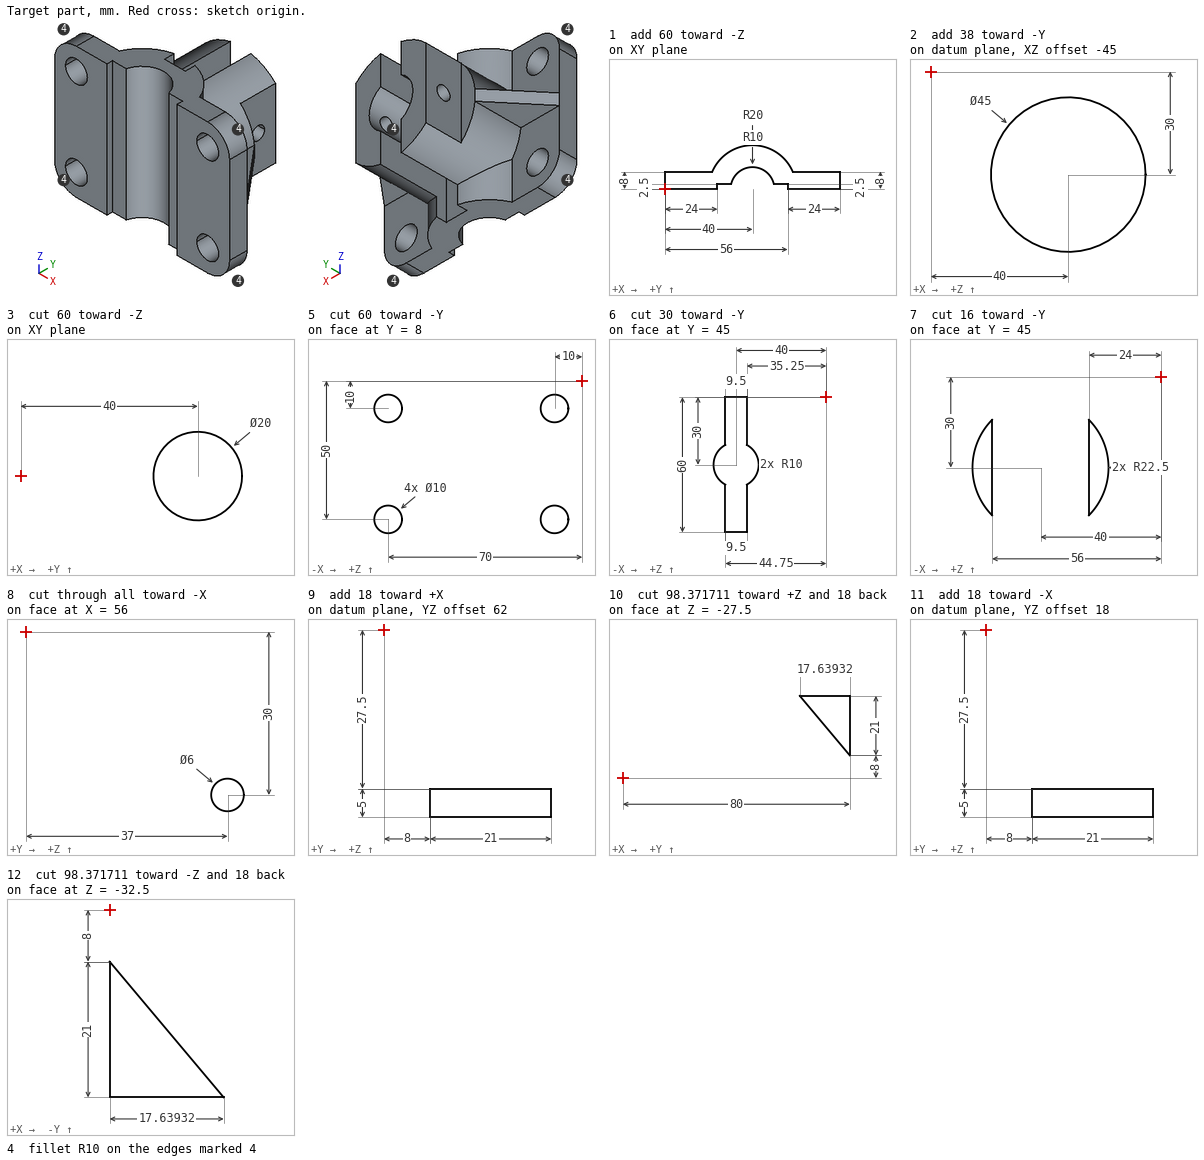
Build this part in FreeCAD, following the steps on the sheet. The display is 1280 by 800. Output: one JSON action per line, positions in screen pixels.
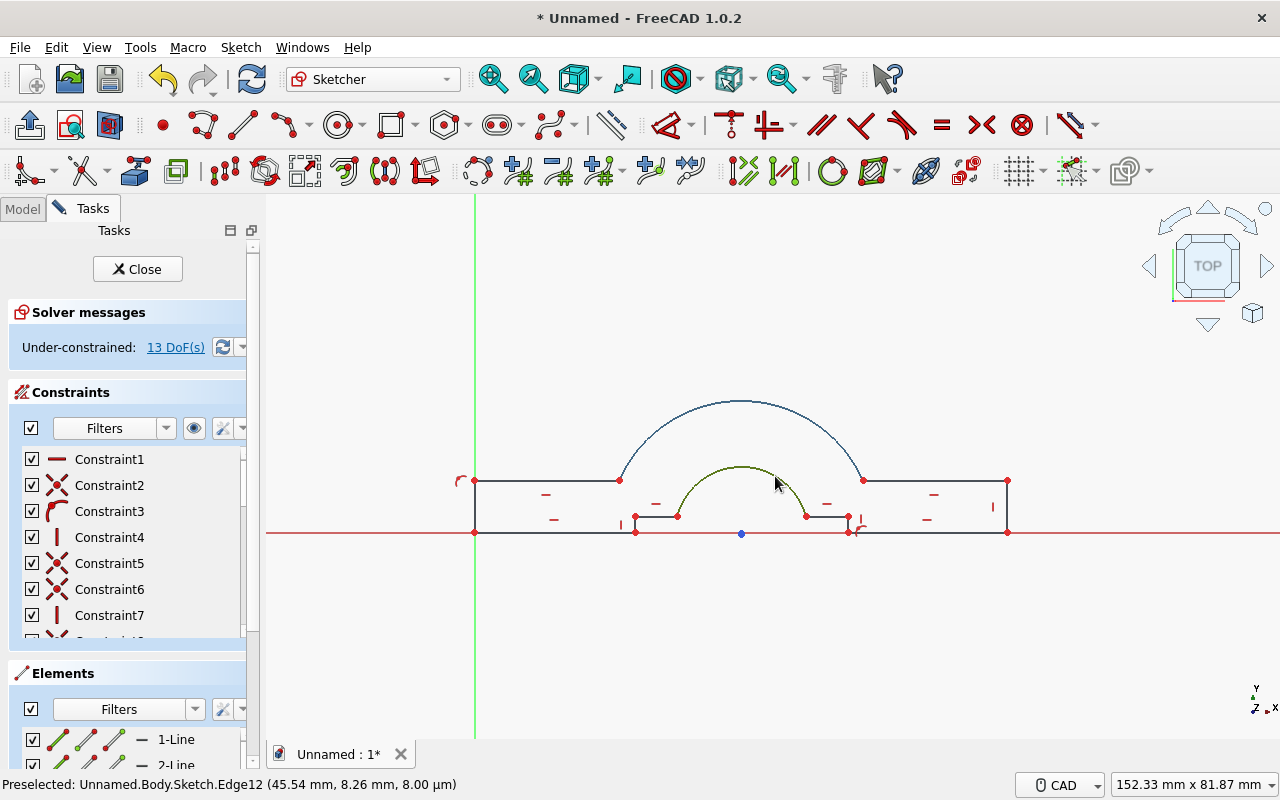
{"action": "left_click", "coordinate": [730, 126]}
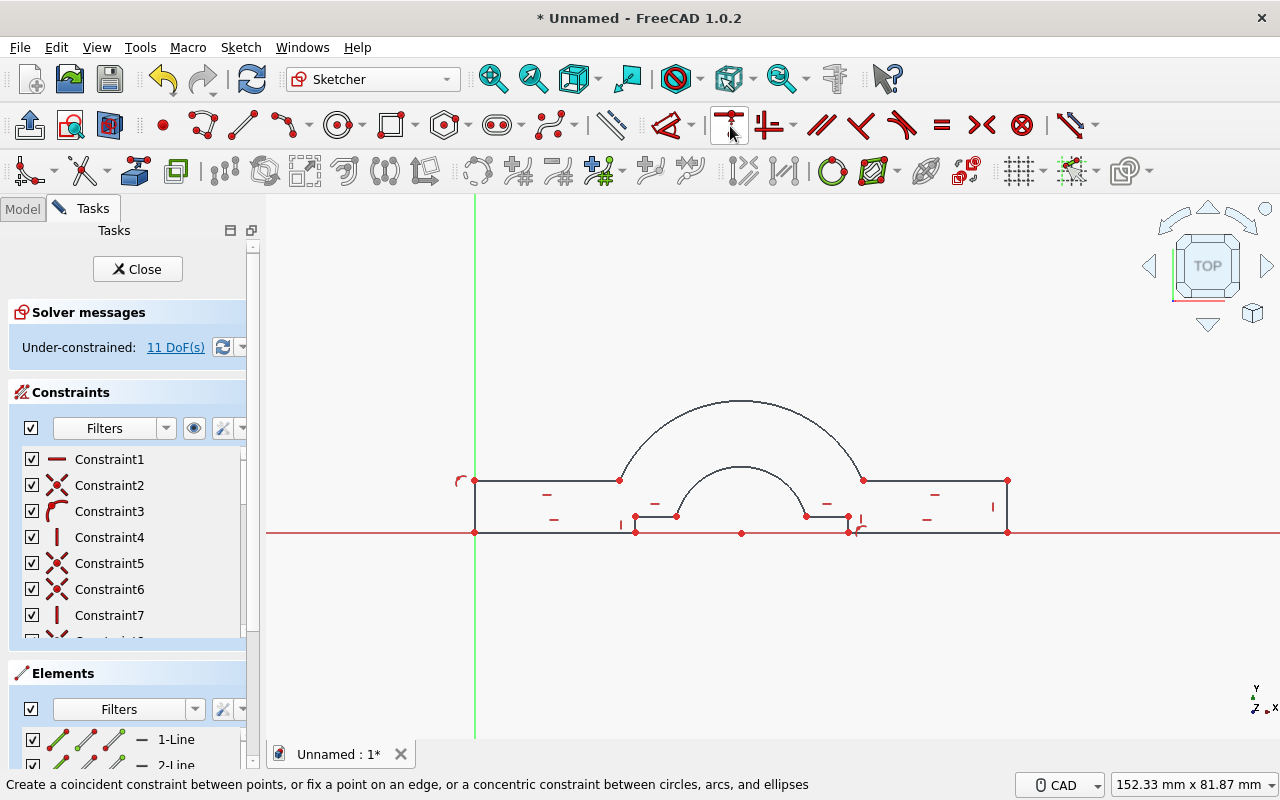
{"action": "left_click", "coordinate": [741, 534]}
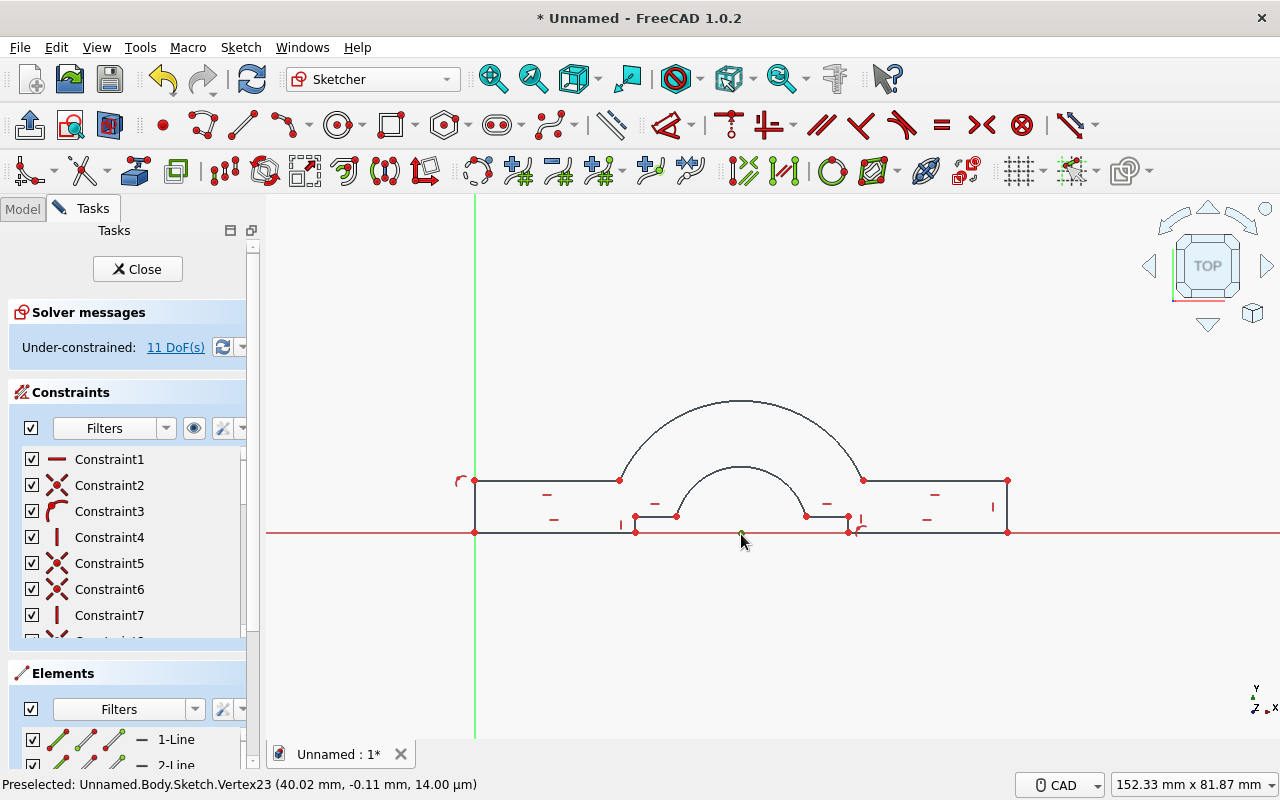
{"action": "left_click", "coordinate": [353, 533]}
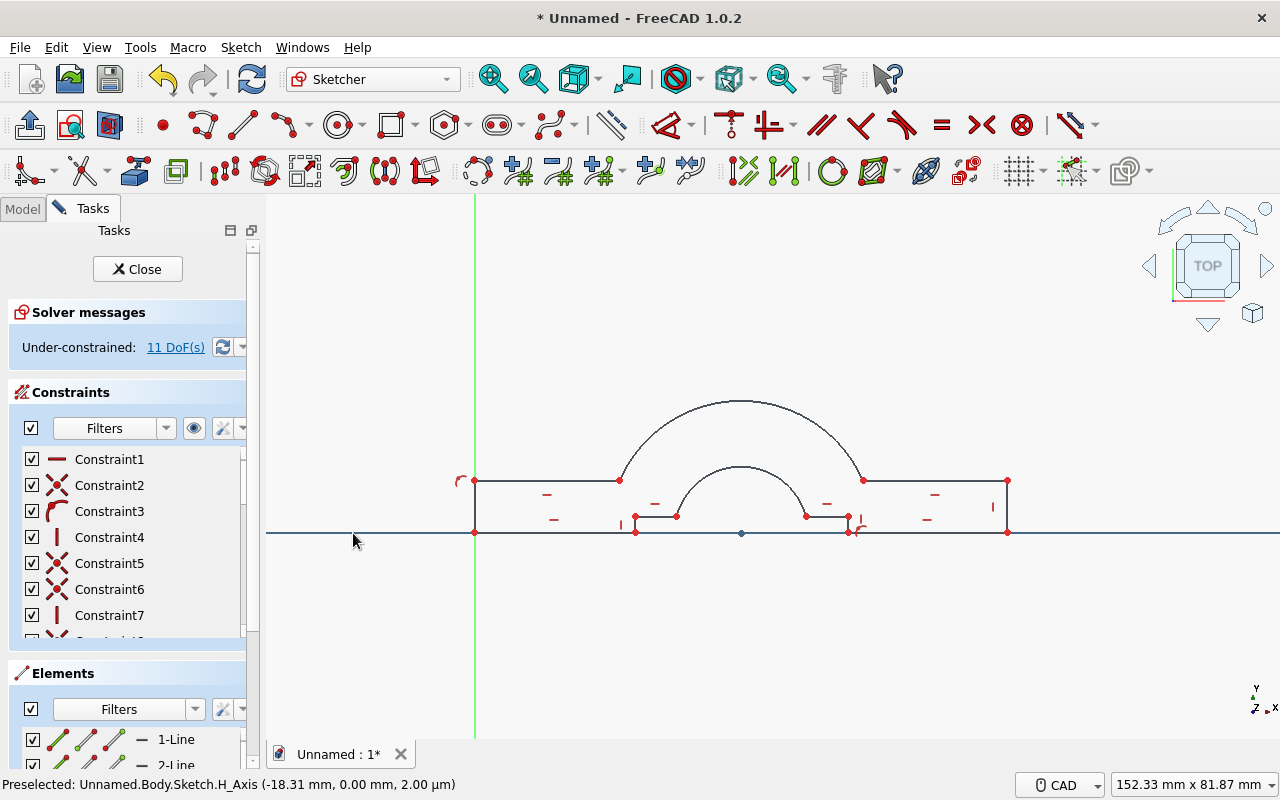
{"action": "left_click", "coordinate": [730, 126]}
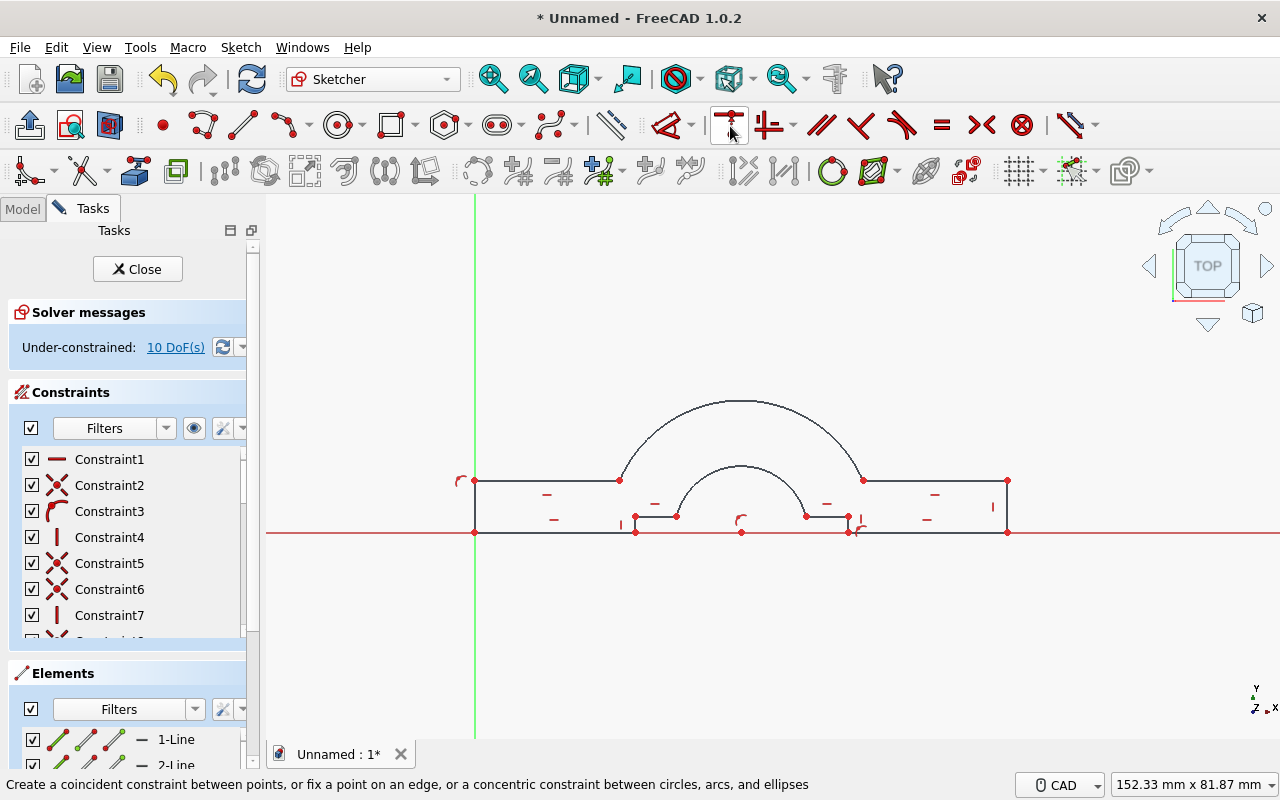
{"action": "left_click", "coordinate": [666, 126]}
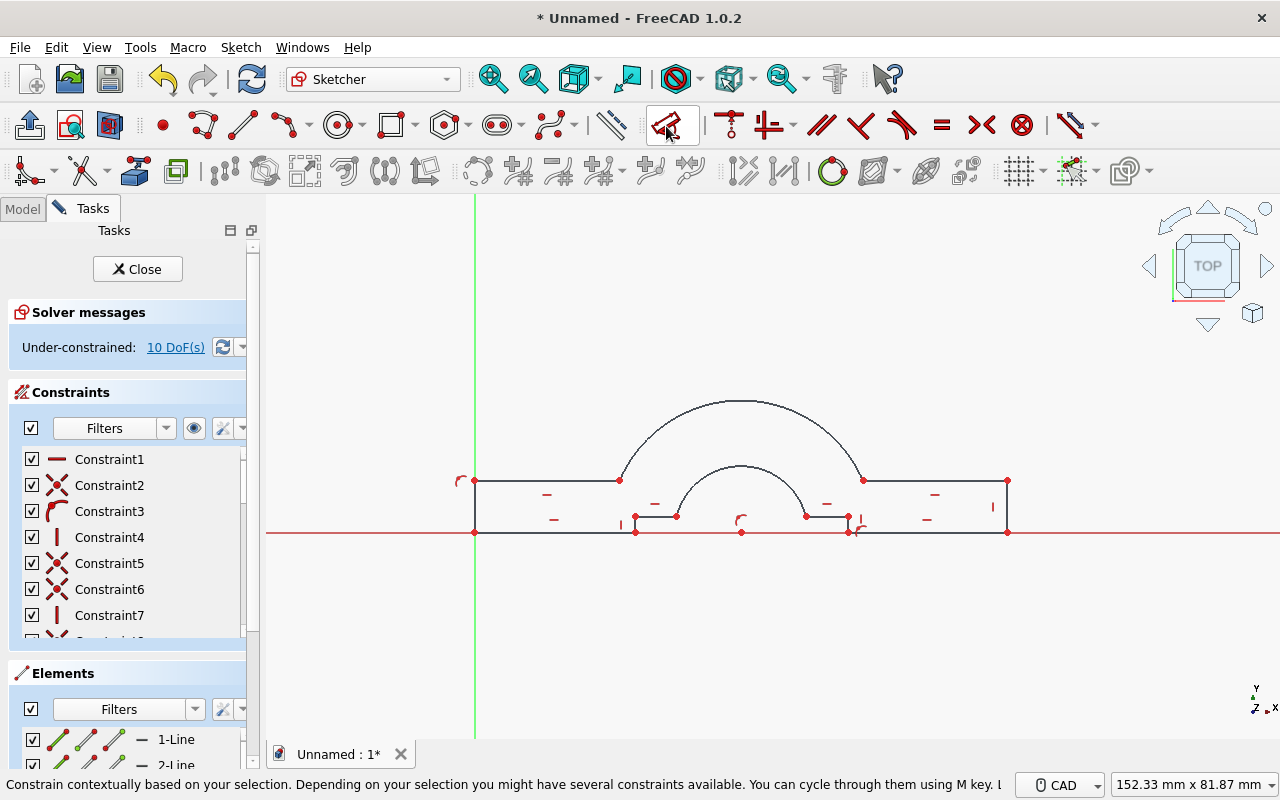
{"action": "left_click", "coordinate": [801, 415]}
{"action": "left_click", "coordinate": [815, 386]}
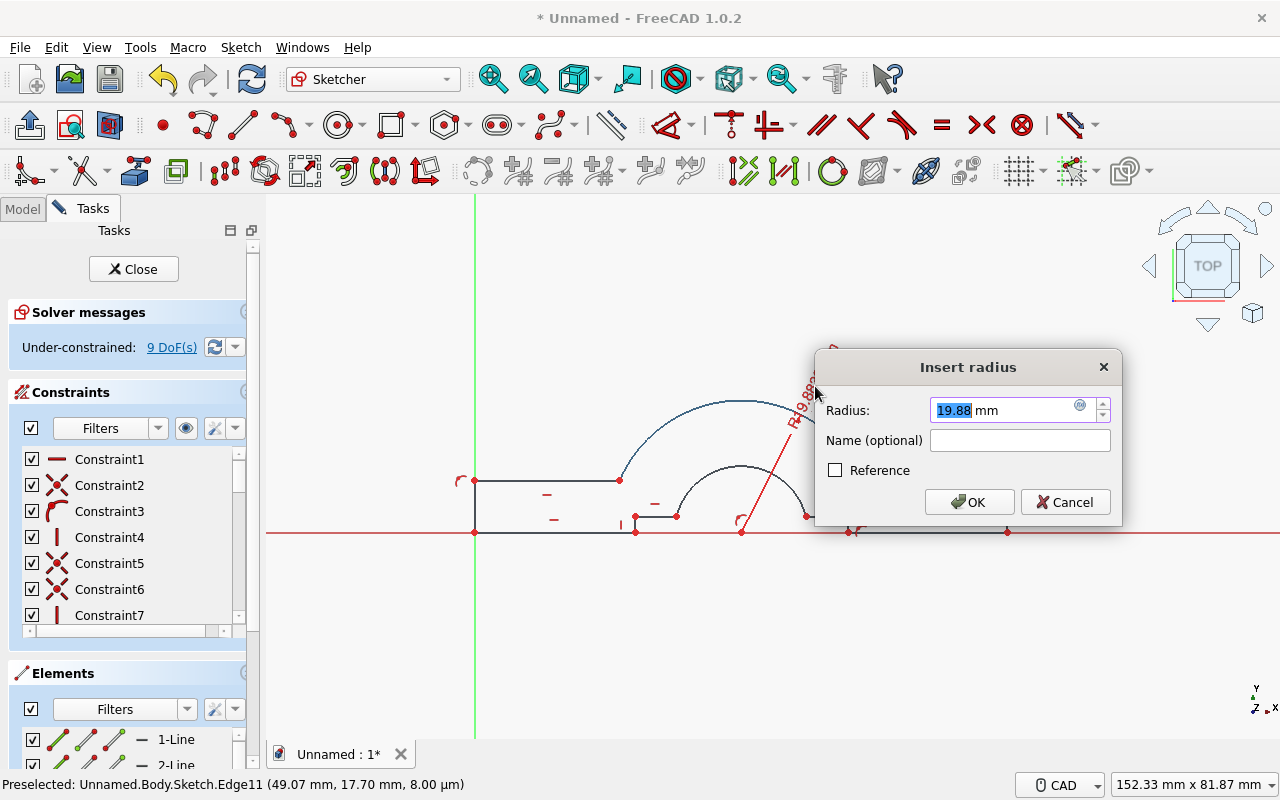
{"action": "type", "text": "20"}
{"action": "key", "text": "Return"}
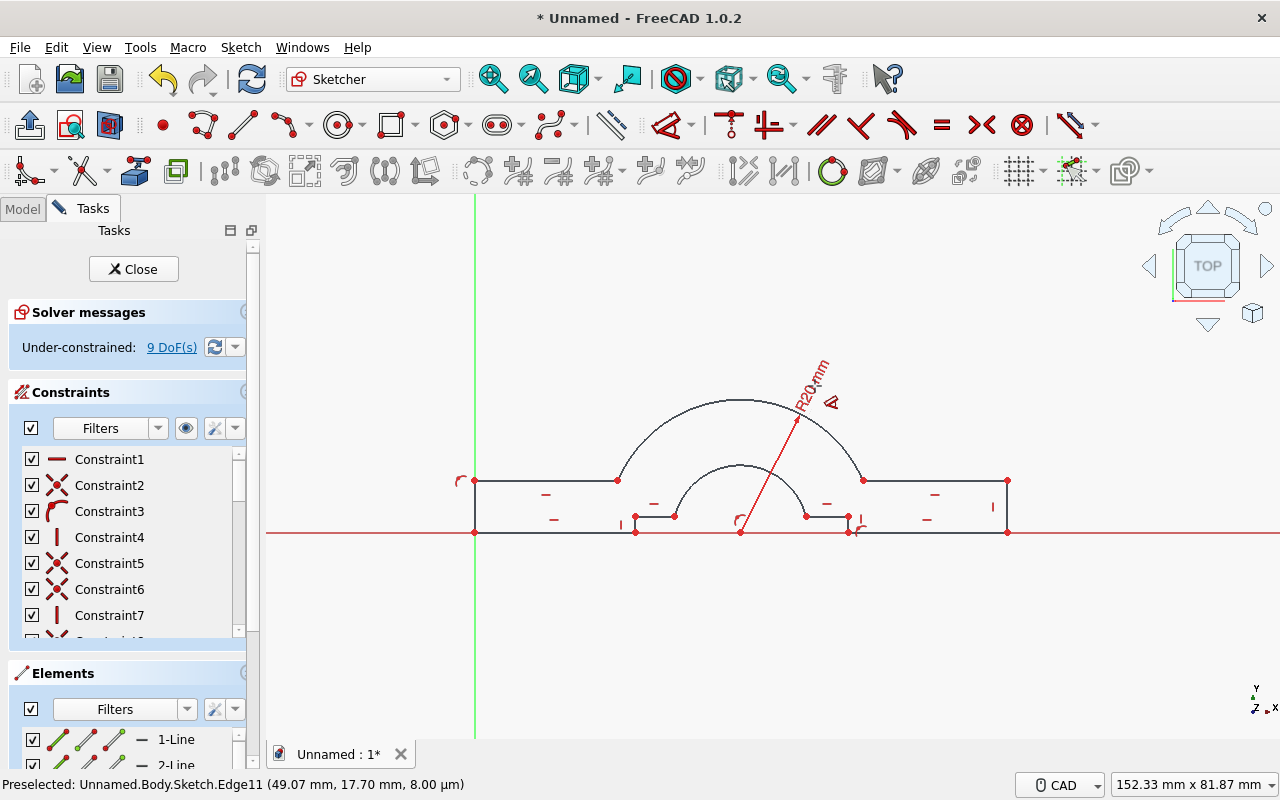
{"action": "left_click", "coordinate": [775, 475]}
{"action": "left_click", "coordinate": [791, 448]}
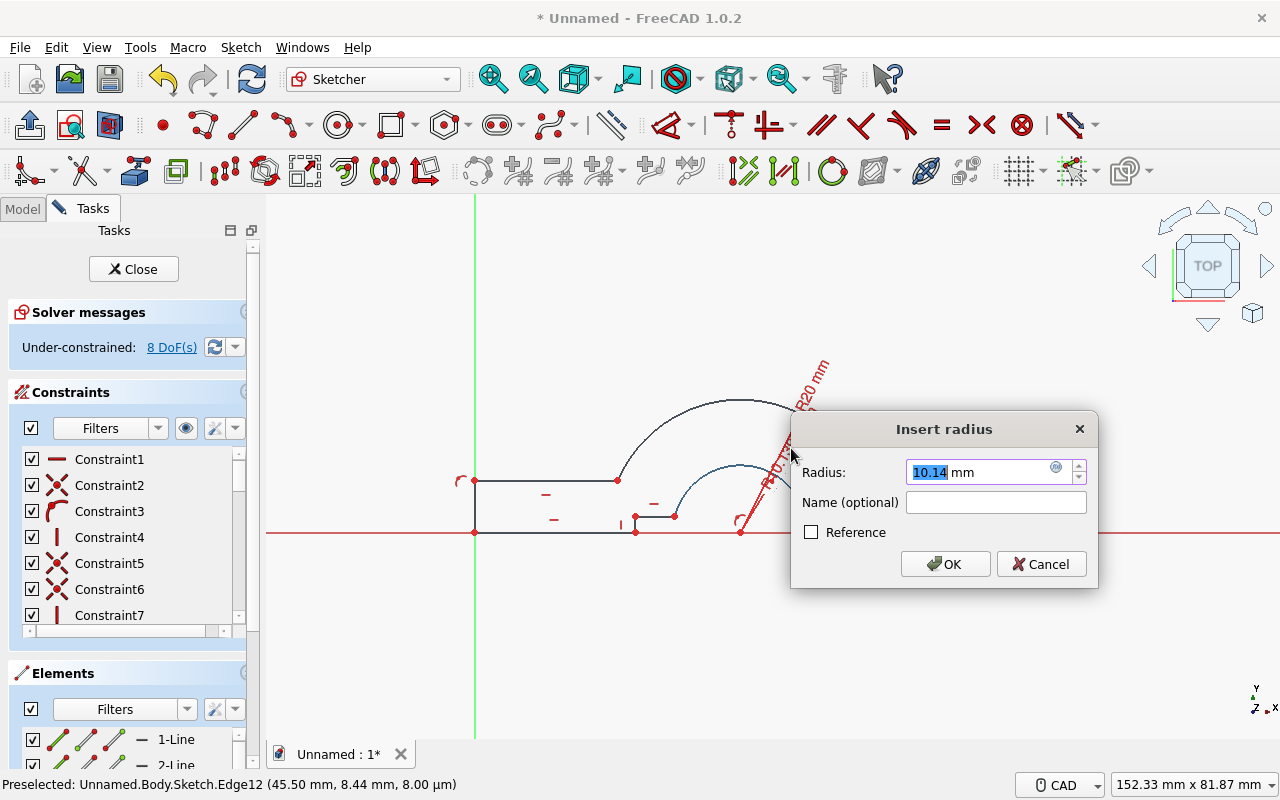
{"action": "type", "text": "10"}
{"action": "key", "text": "Return"}